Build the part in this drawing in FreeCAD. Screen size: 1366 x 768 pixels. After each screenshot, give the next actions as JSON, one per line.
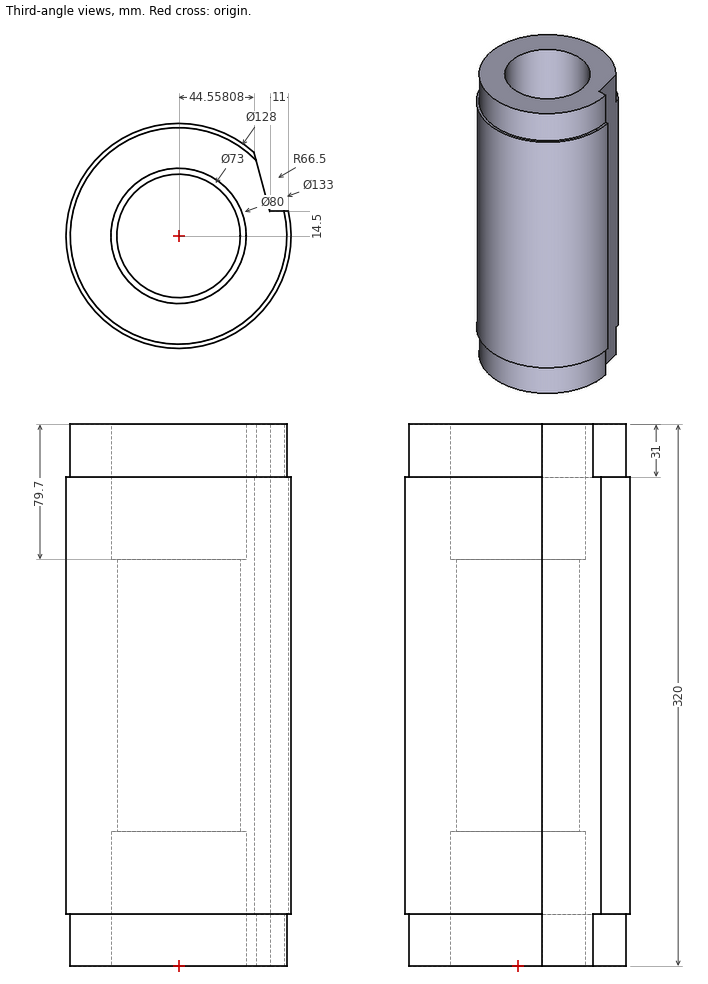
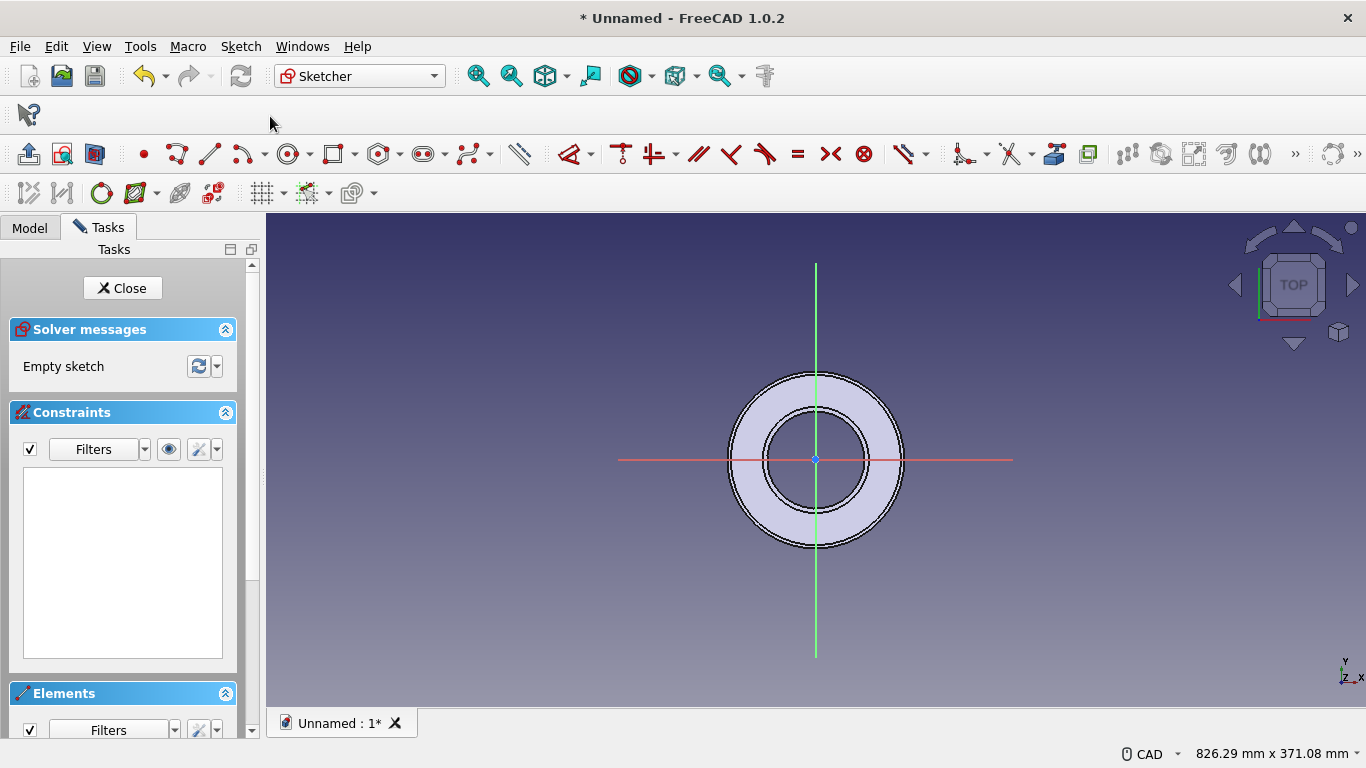
{"action": "scroll", "coordinate": [887, 419], "scroll_direction": "up", "scroll_amount": 8}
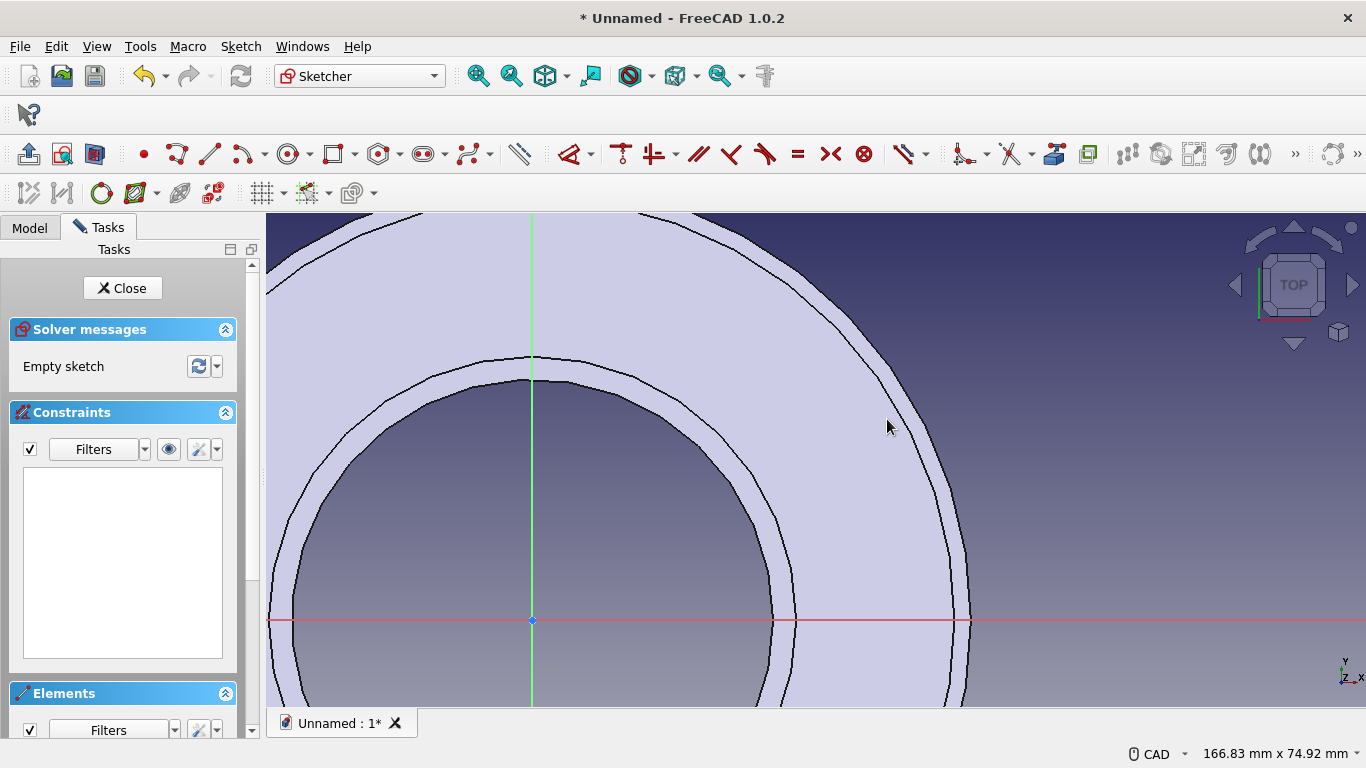
{"action": "left_click", "coordinate": [177, 154]}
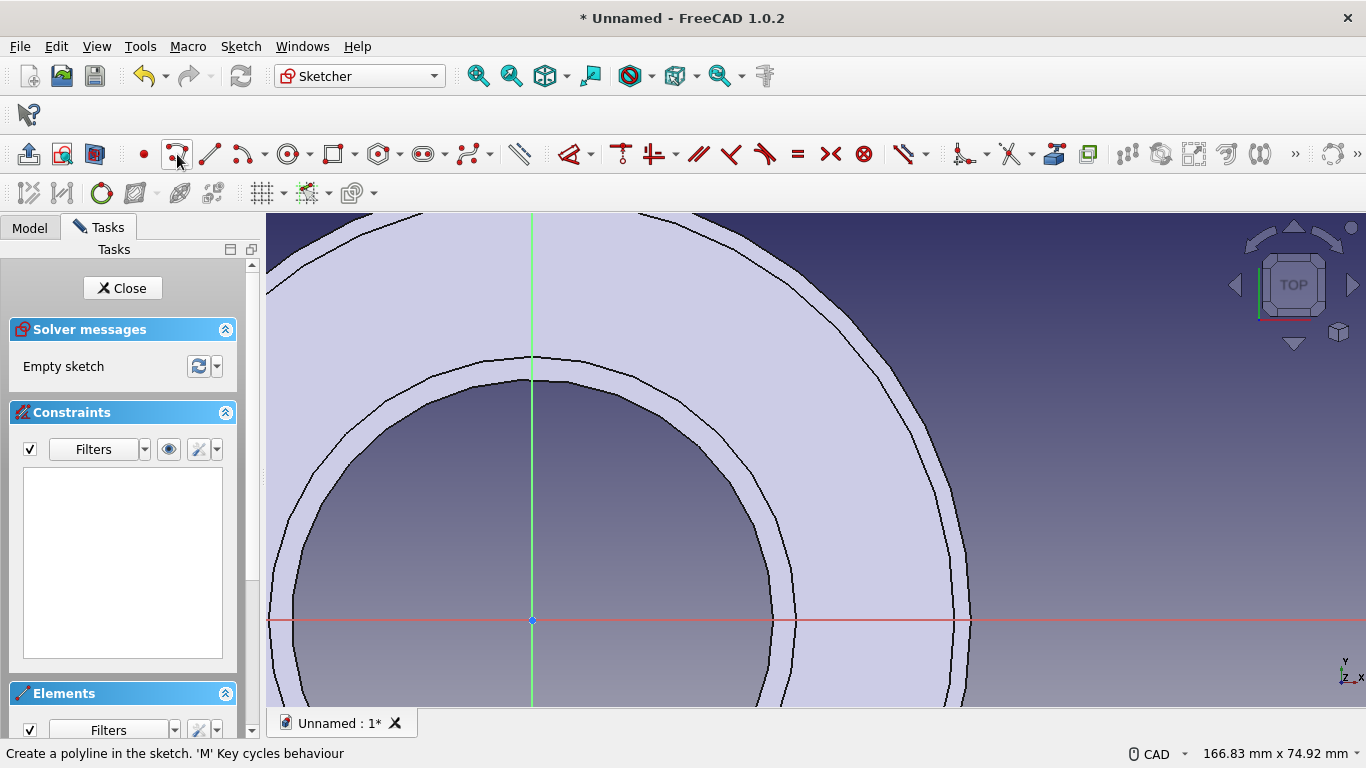
{"action": "left_click", "coordinate": [826, 295]}
{"action": "left_click", "coordinate": [888, 525]}
{"action": "left_click", "coordinate": [960, 525]}
{"action": "right_click", "coordinate": [960, 525]}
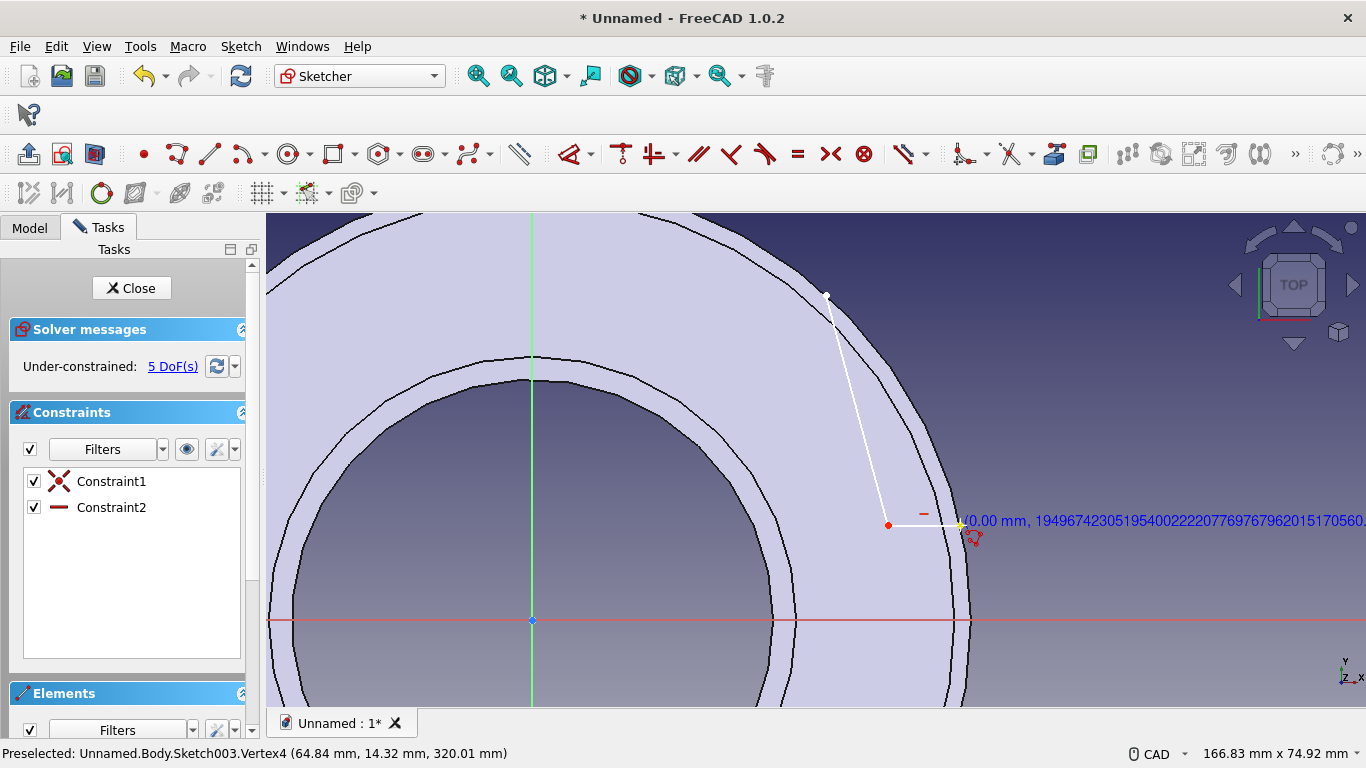
{"action": "left_click", "coordinate": [264, 154]}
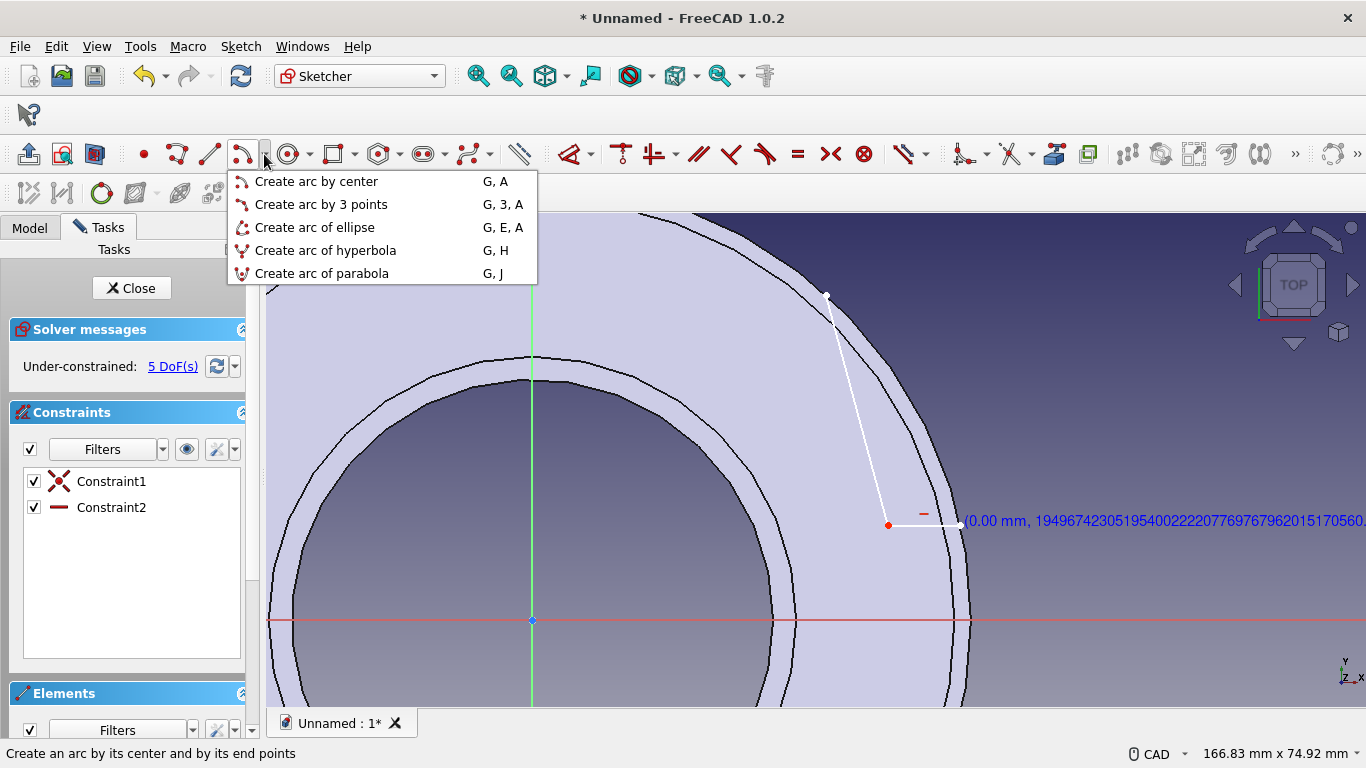
{"action": "left_click", "coordinate": [382, 204]}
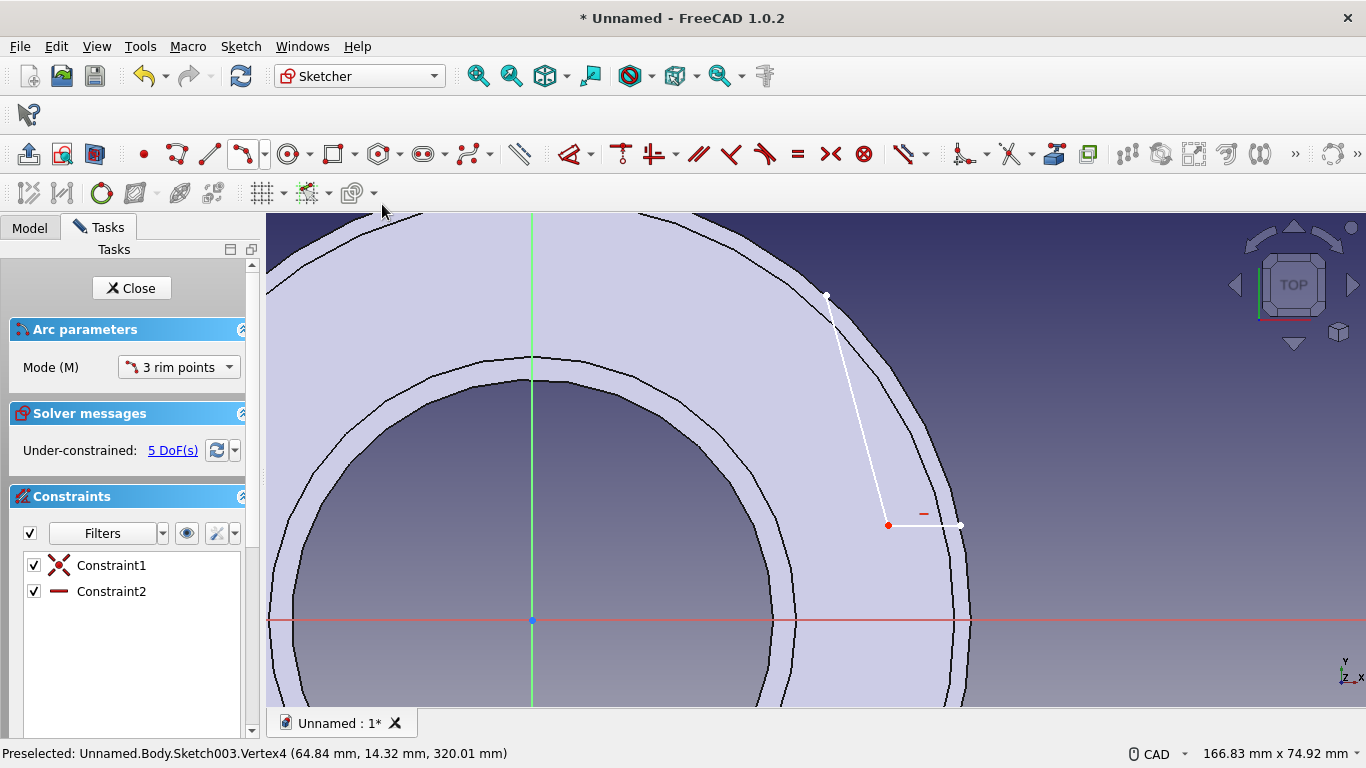
{"action": "left_click", "coordinate": [960, 526]}
{"action": "left_click", "coordinate": [826, 296]}
{"action": "left_click", "coordinate": [911, 399]}
{"action": "key", "text": "Escape"}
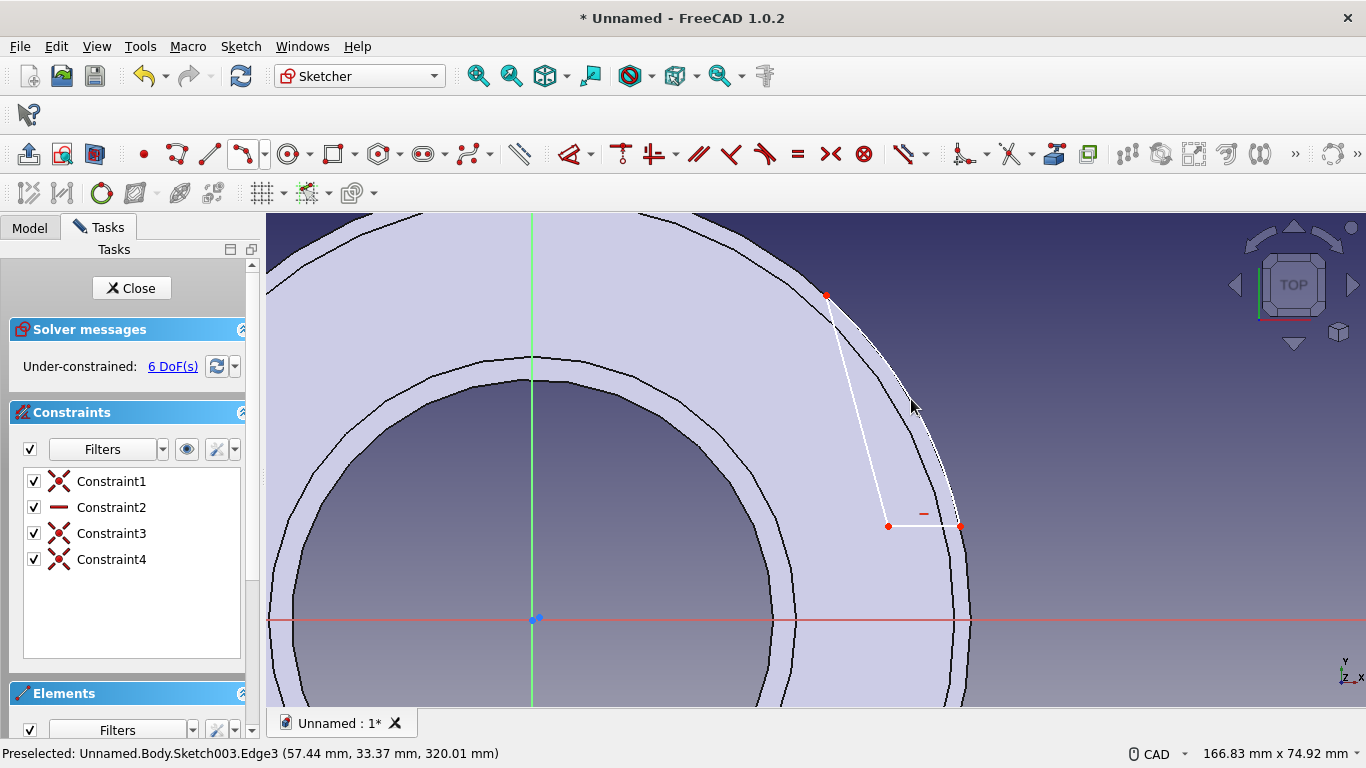
{"action": "left_click_drag", "start_coordinate": [522, 607], "coordinate": [549, 630]}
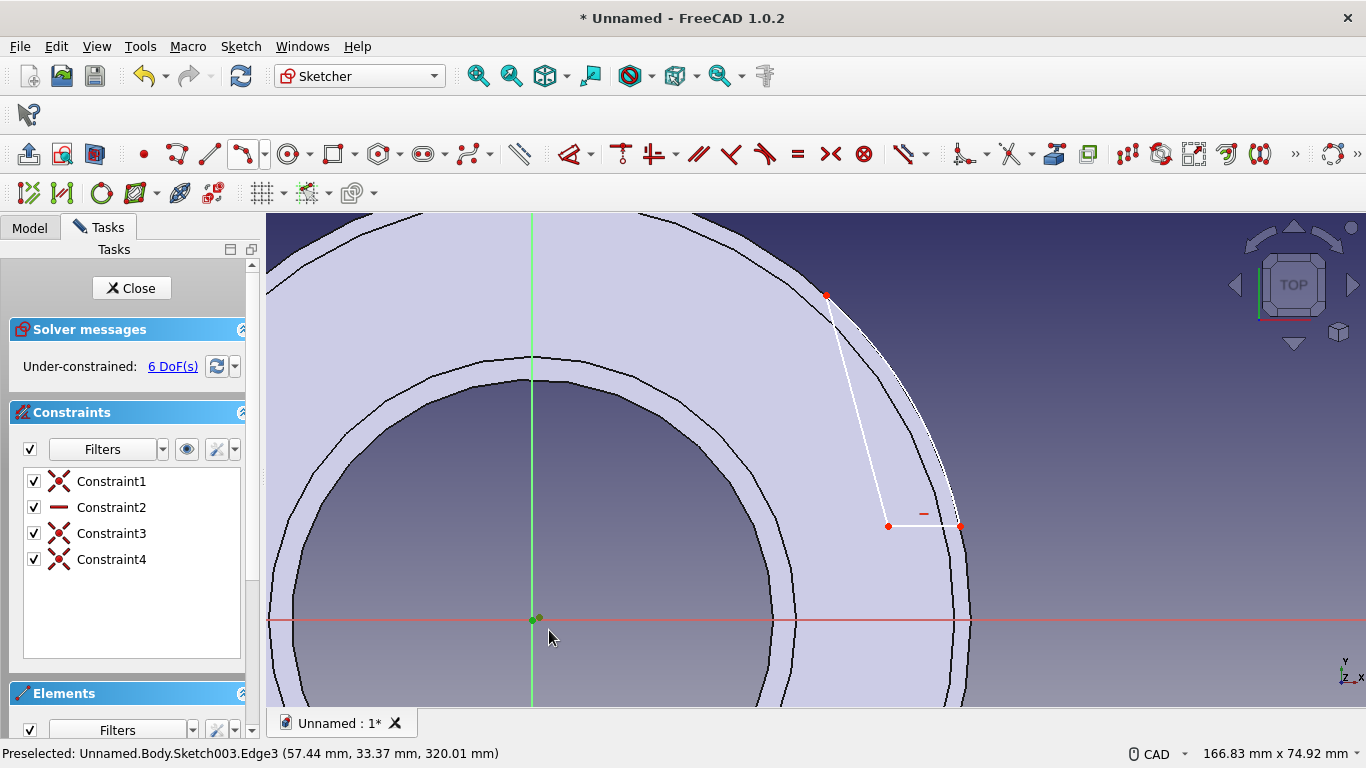
{"action": "left_click", "coordinate": [621, 154]}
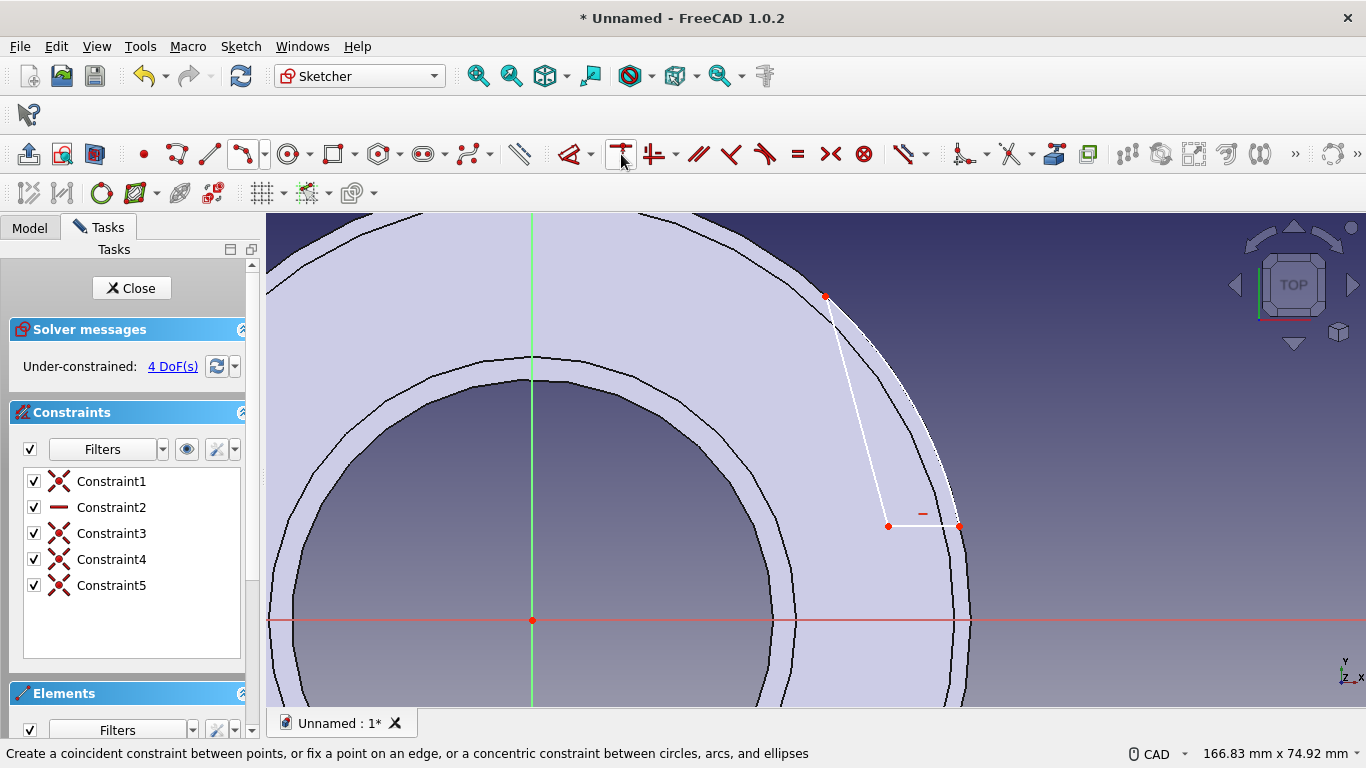
{"action": "left_click", "coordinate": [568, 154]}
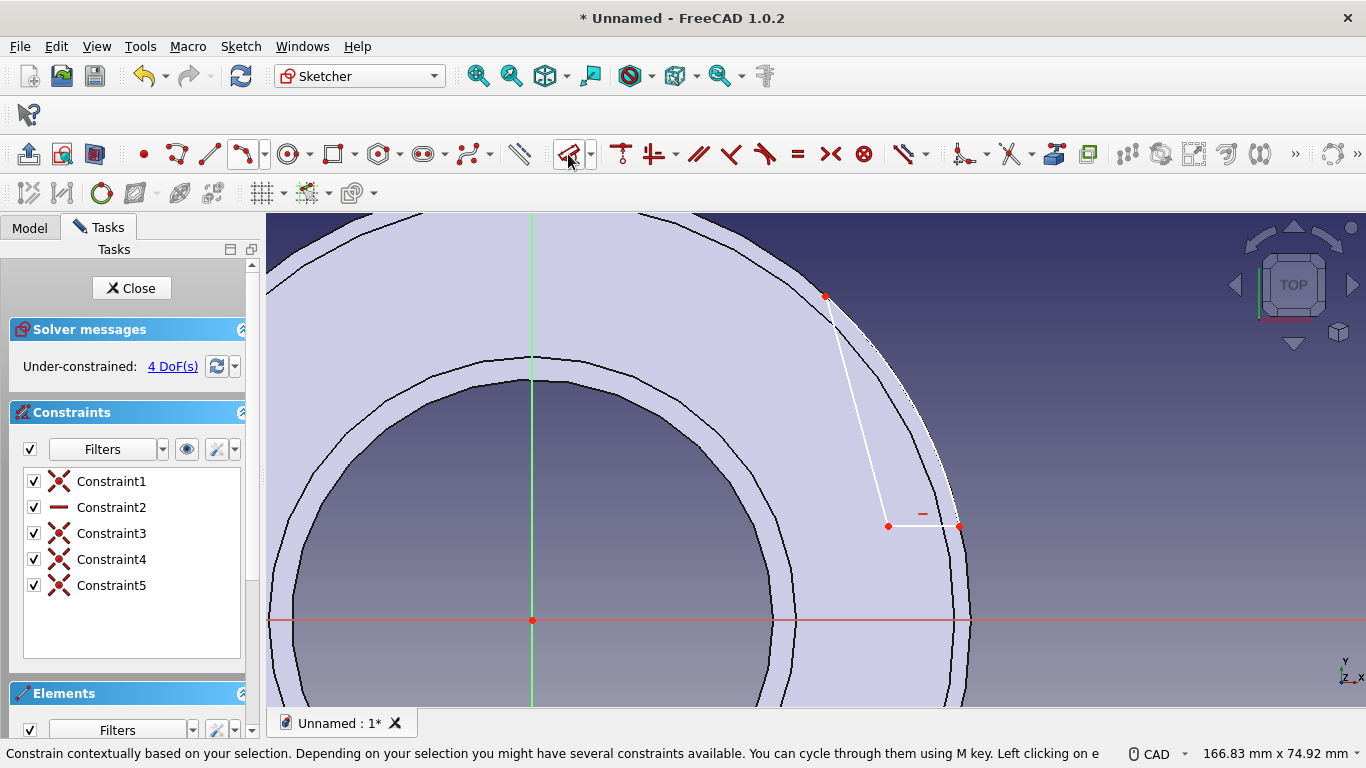
{"action": "left_click", "coordinate": [935, 449]}
{"action": "left_click", "coordinate": [964, 436]}